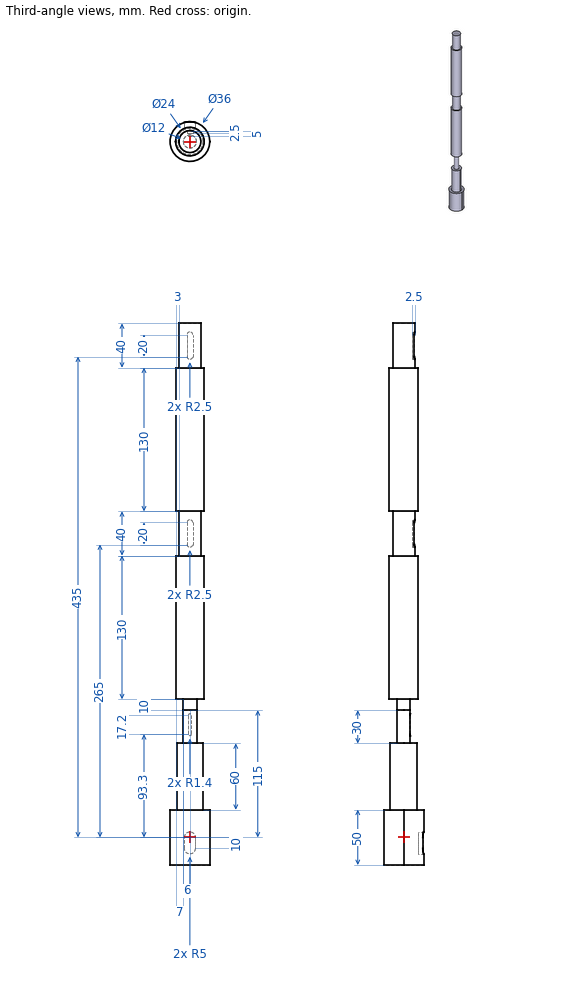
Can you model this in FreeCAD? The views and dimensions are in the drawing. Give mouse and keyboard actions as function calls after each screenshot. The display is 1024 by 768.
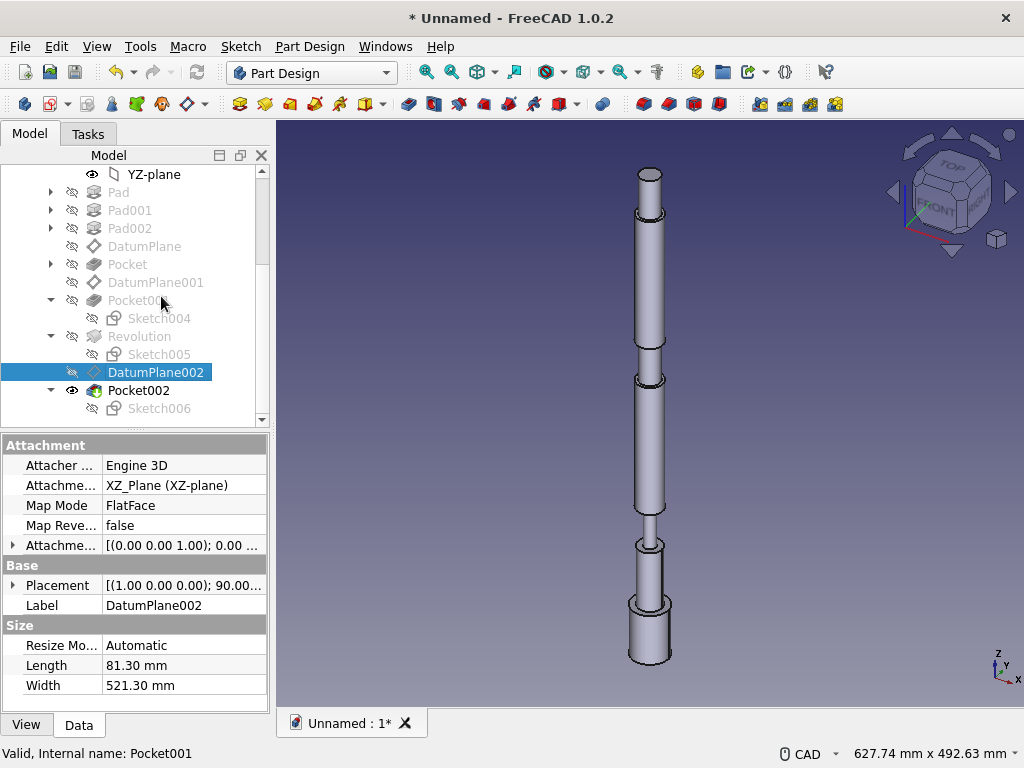
scroll(161, 296, up, 15)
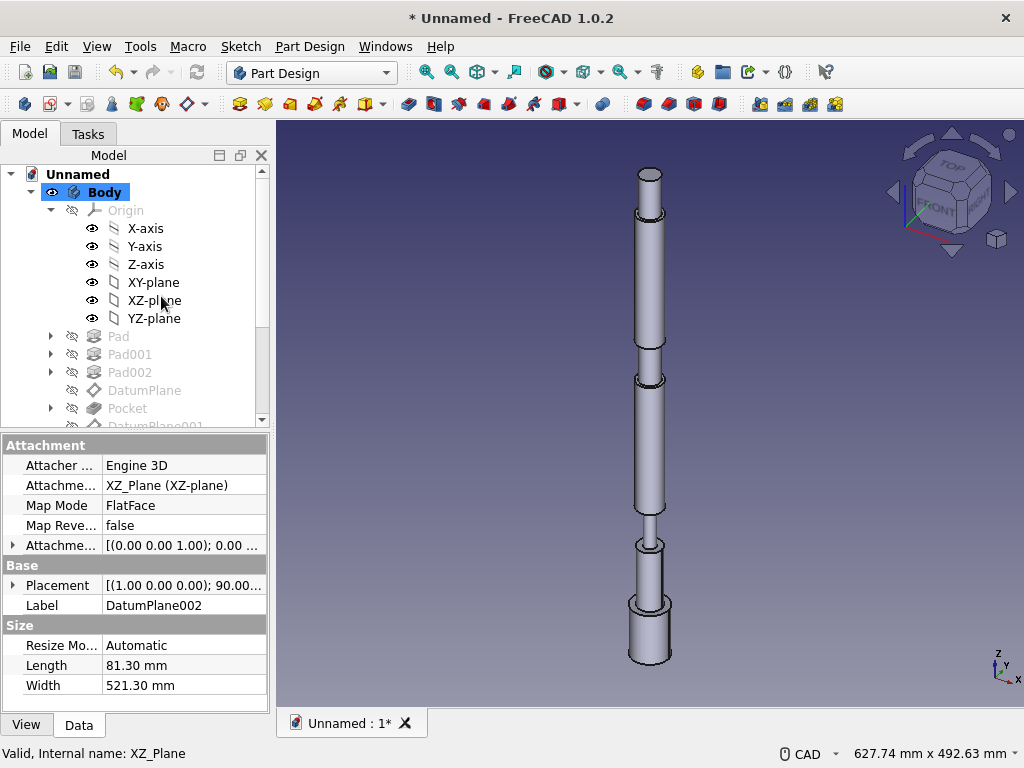
click(137, 300)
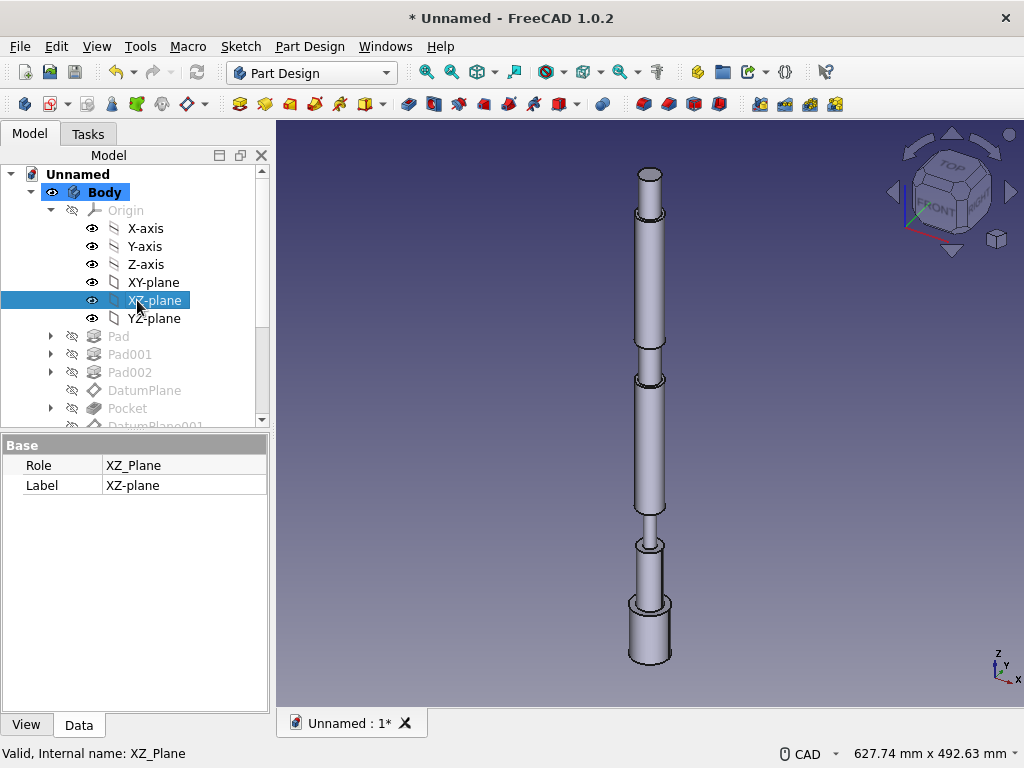
click(186, 104)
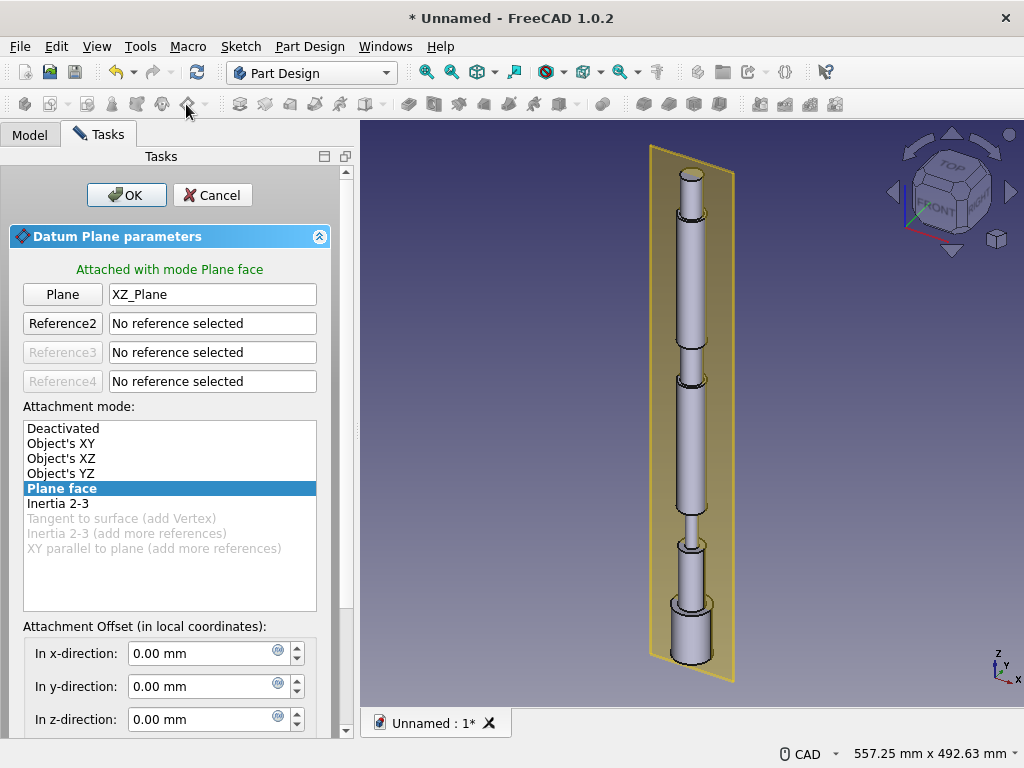
triple_click(210, 720)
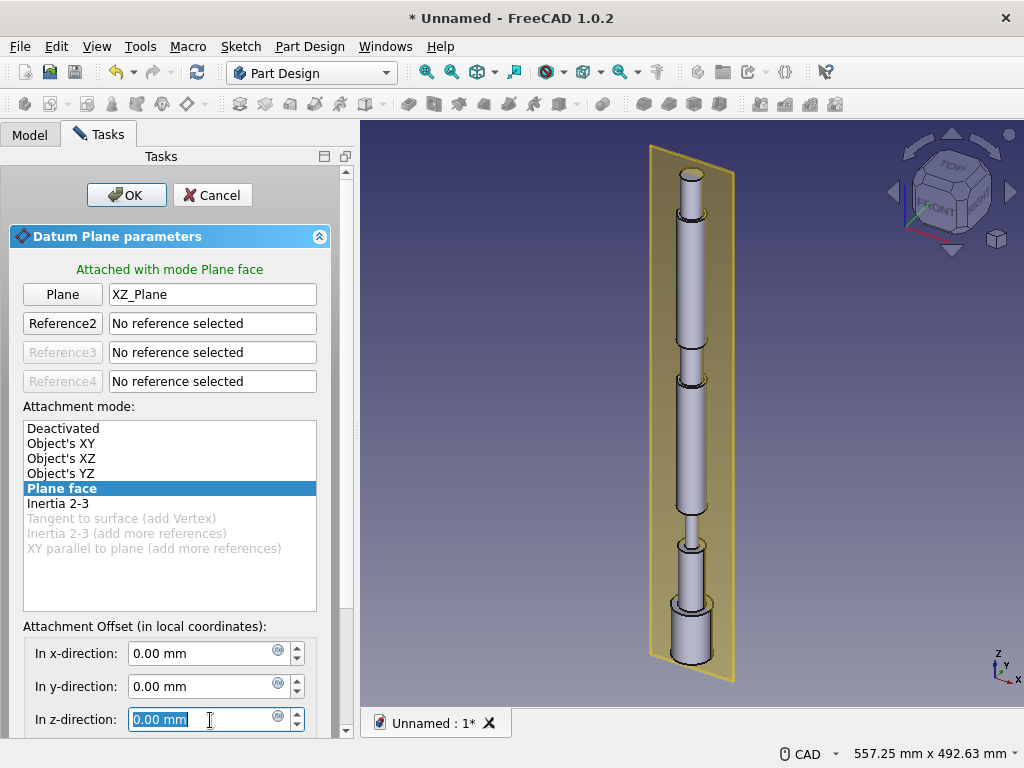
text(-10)
key(Tab)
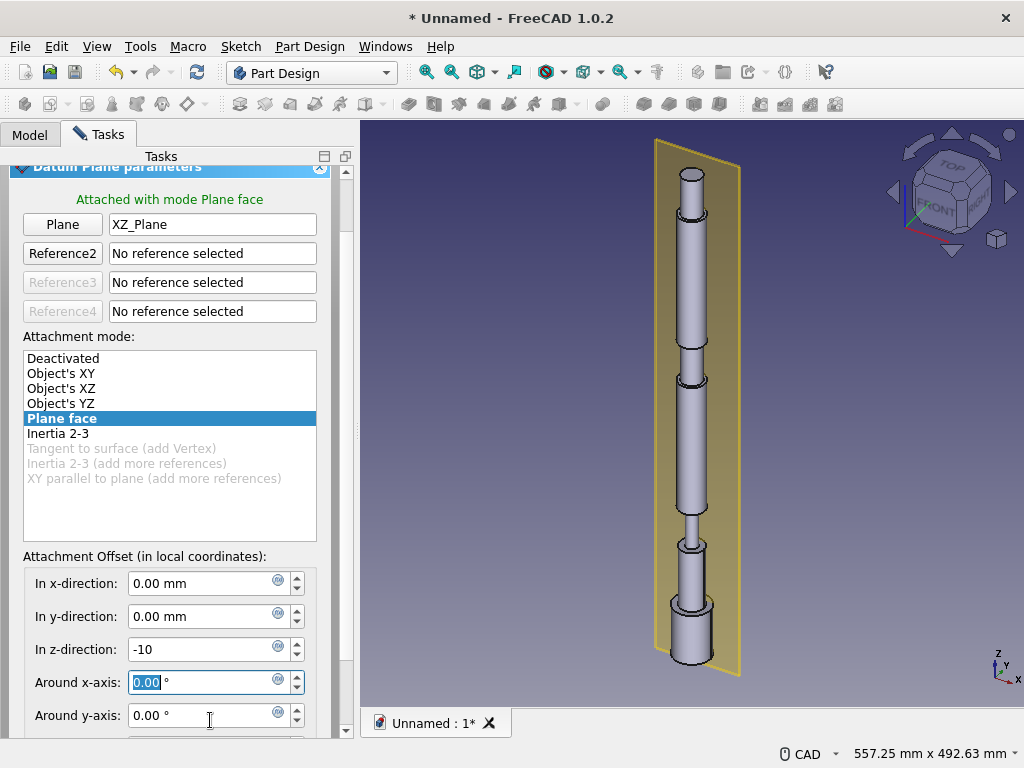
scroll(346, 452, up, 2)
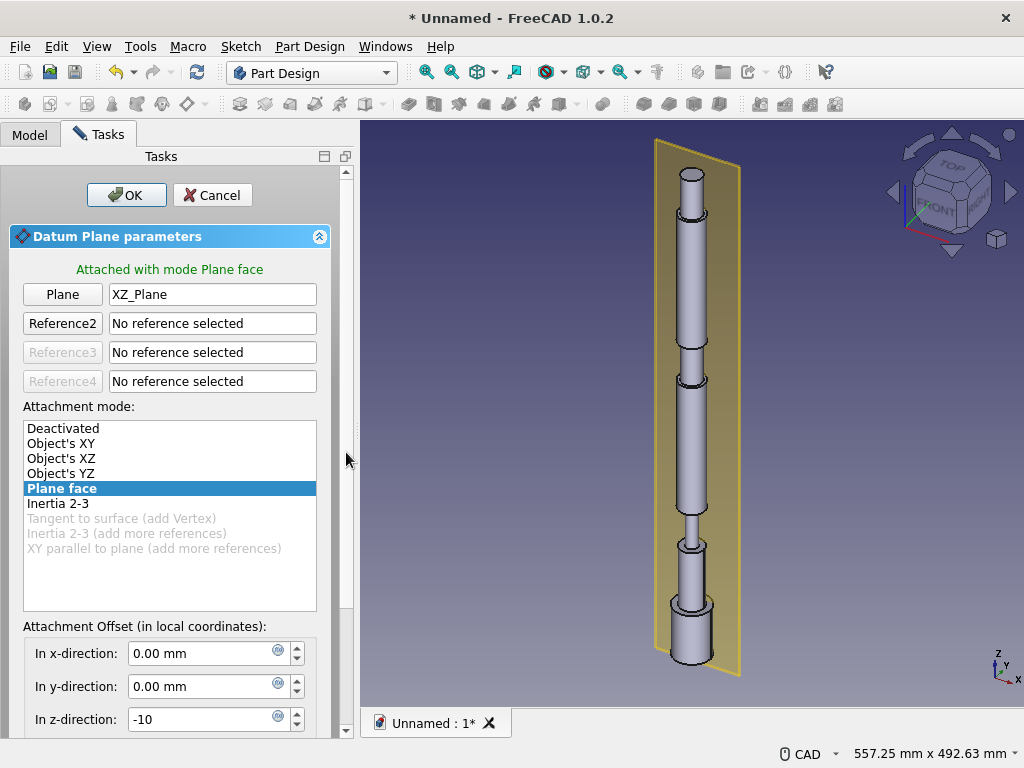
click(127, 195)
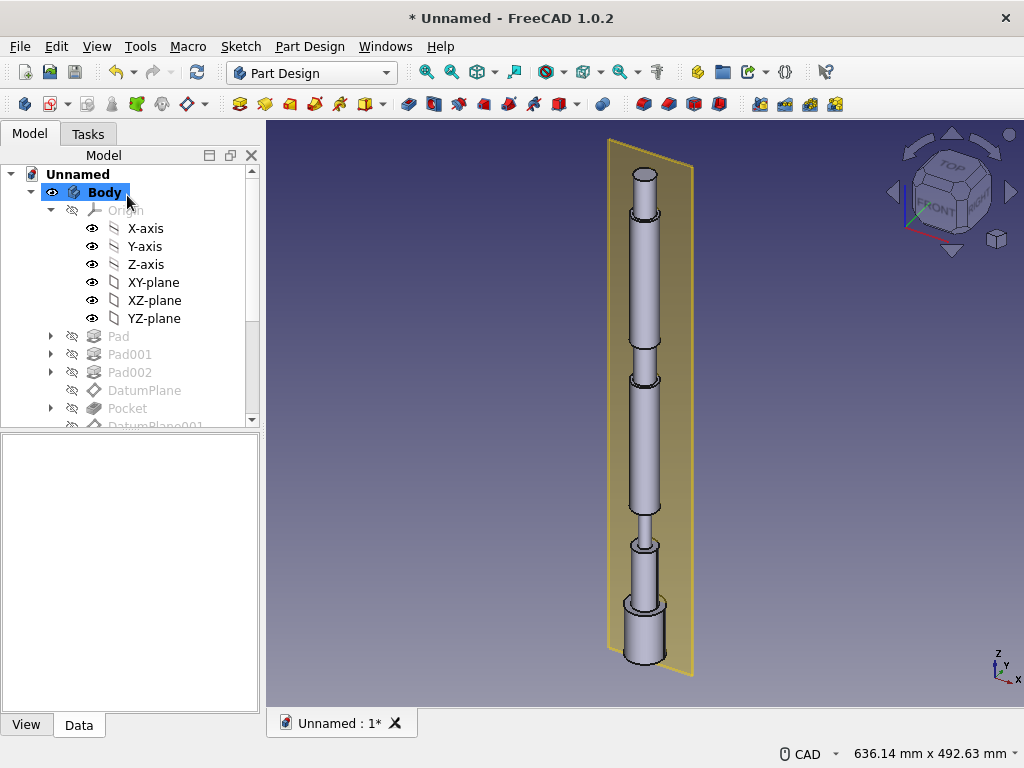
scroll(101, 296, down, 3)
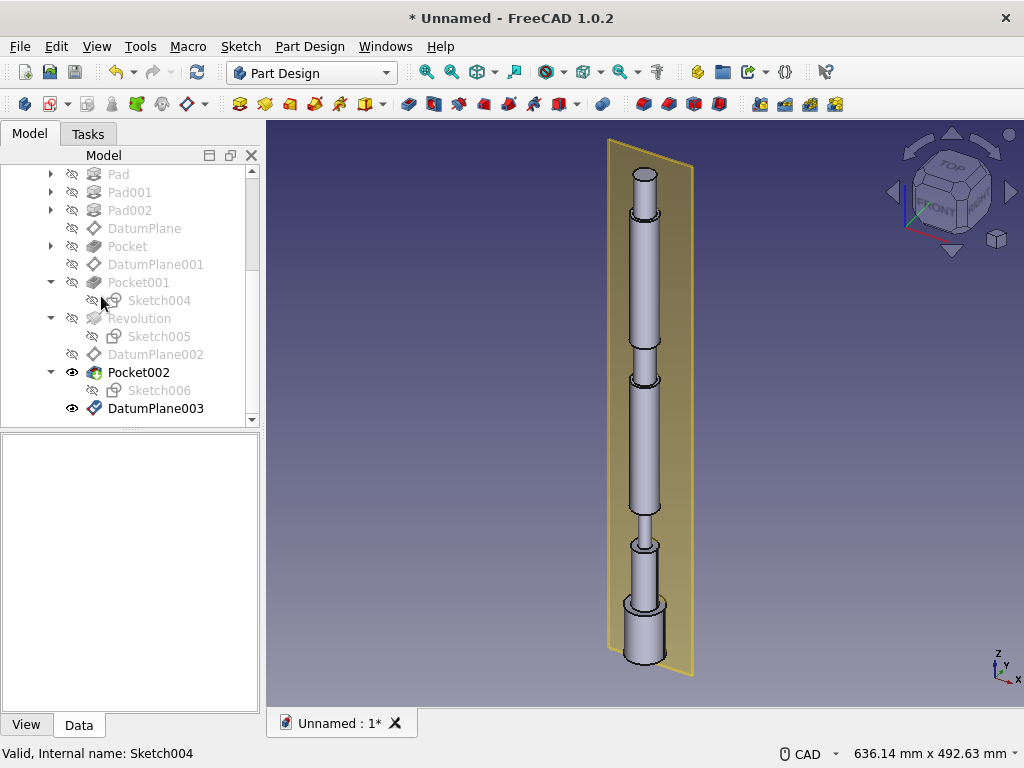
click(117, 408)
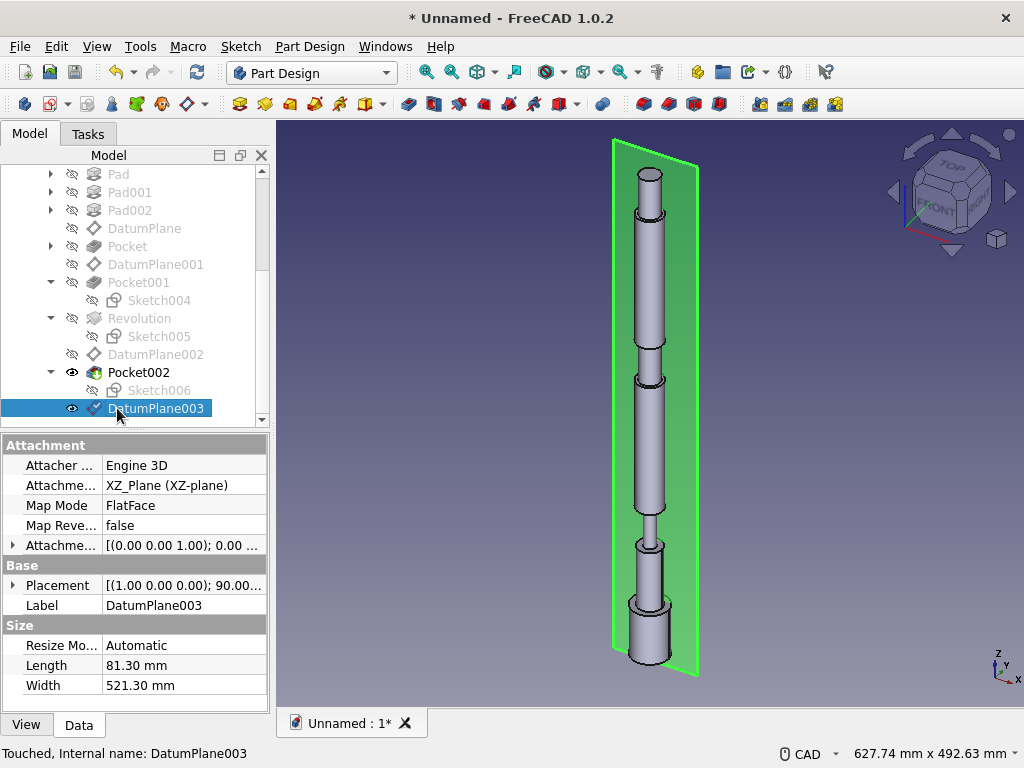
click(50, 104)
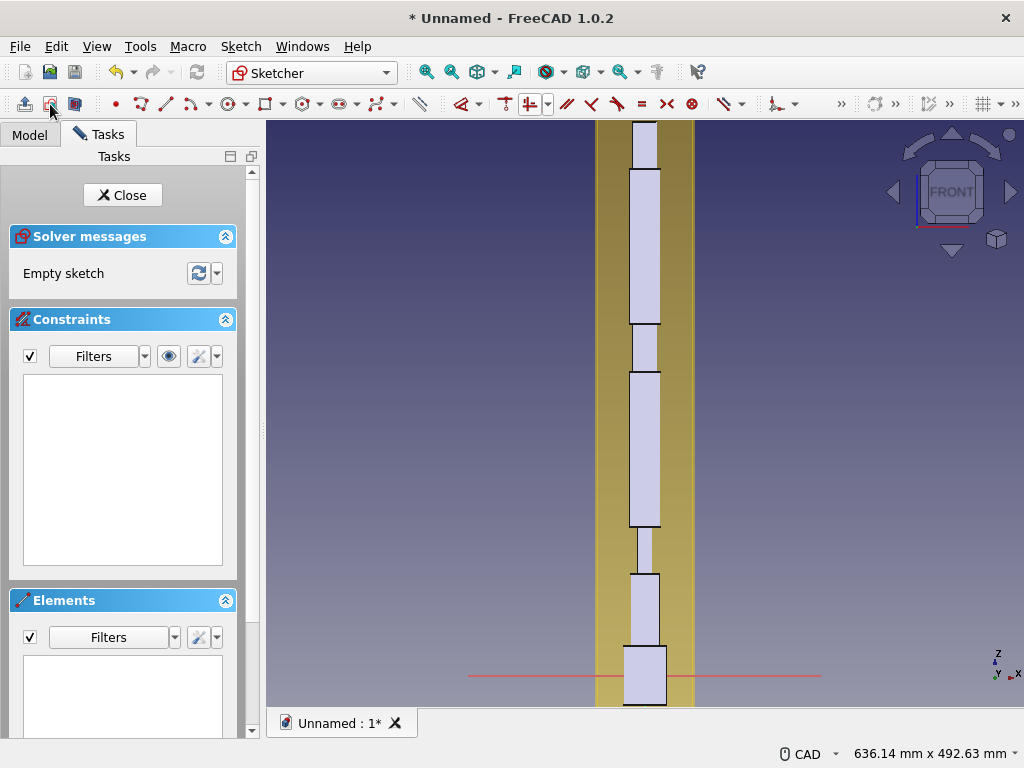
click(75, 104)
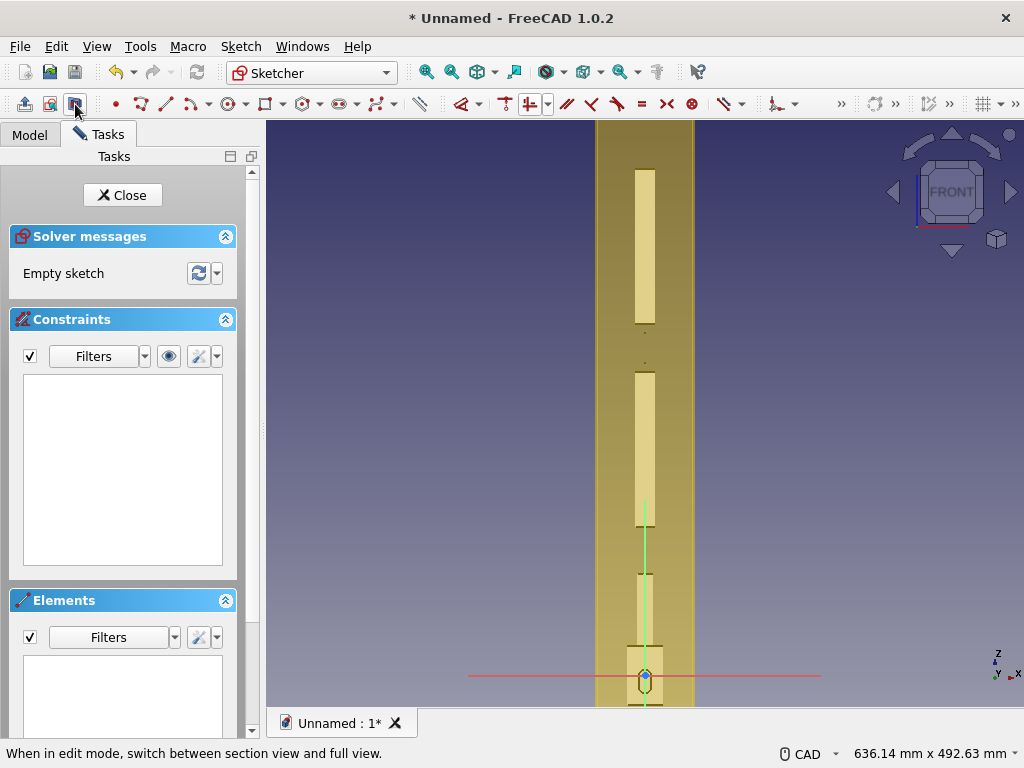
scroll(576, 414, down, 5)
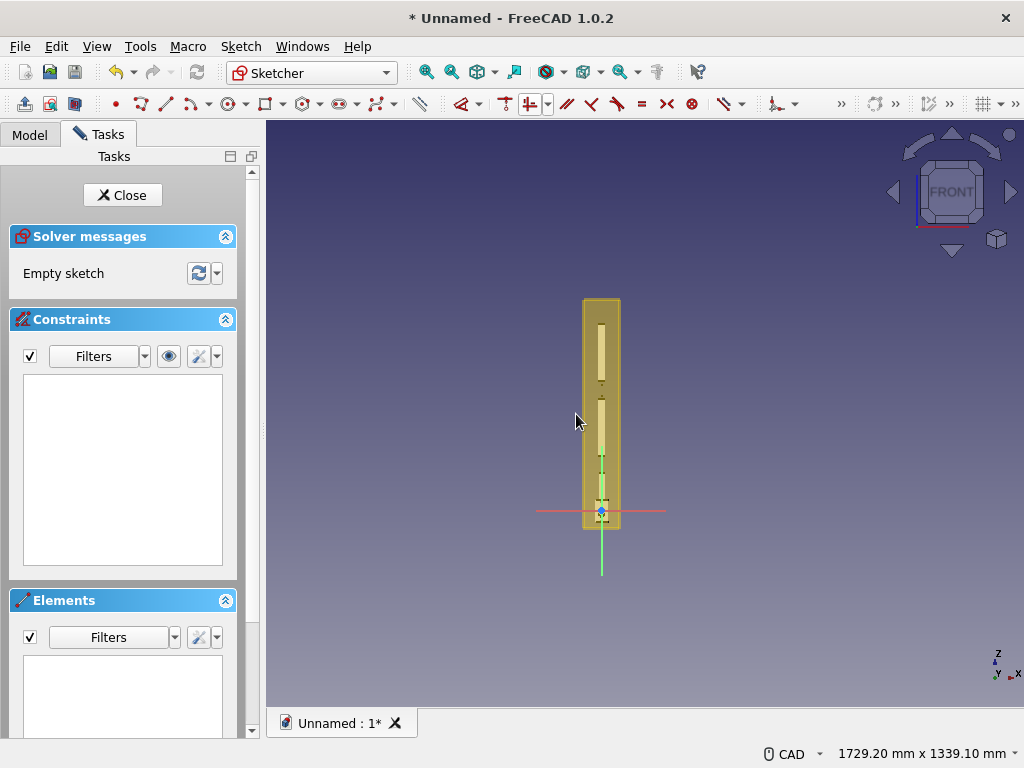
scroll(603, 310, up, 15)